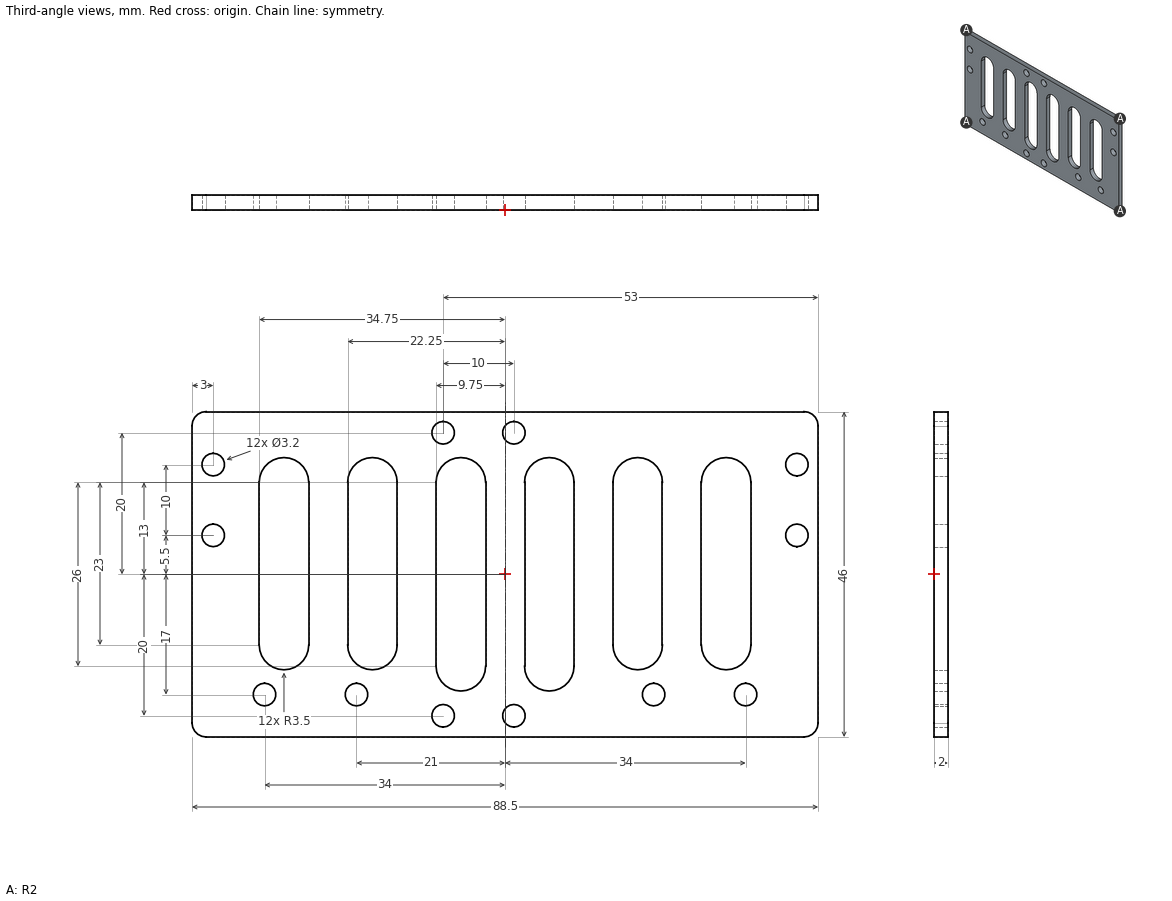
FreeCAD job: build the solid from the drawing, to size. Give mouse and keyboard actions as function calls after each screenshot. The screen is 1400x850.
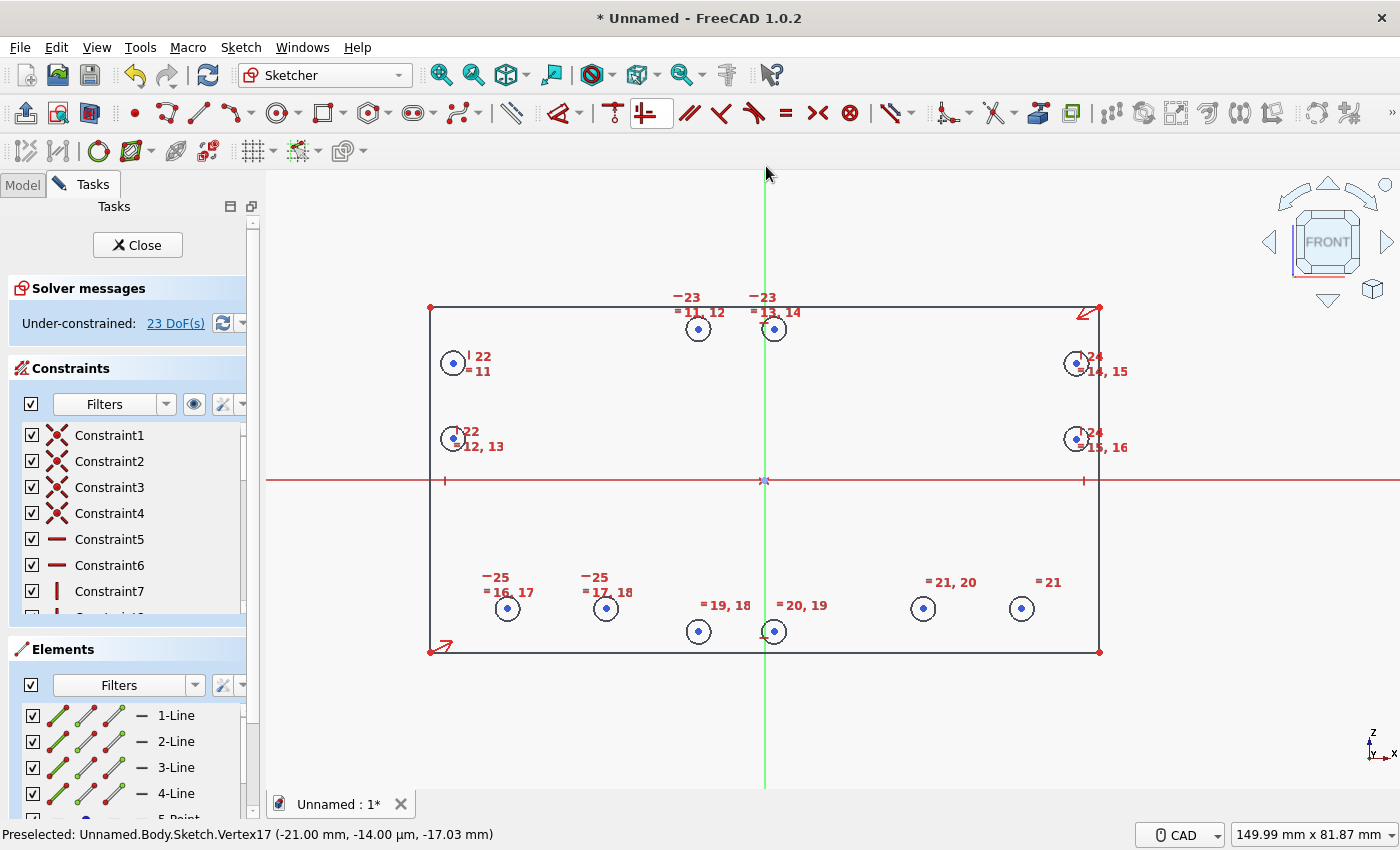
click(698, 329)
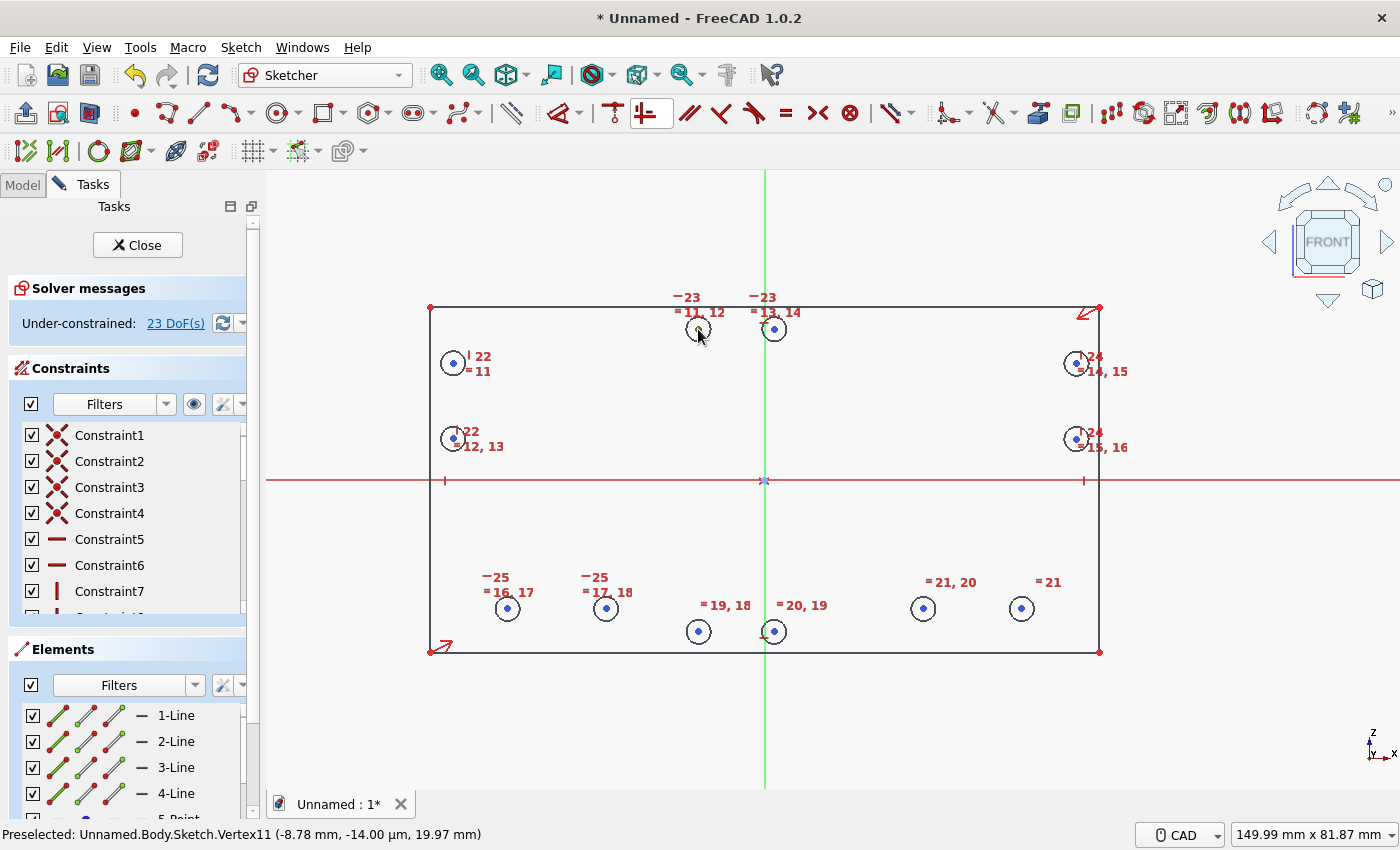
click(699, 632)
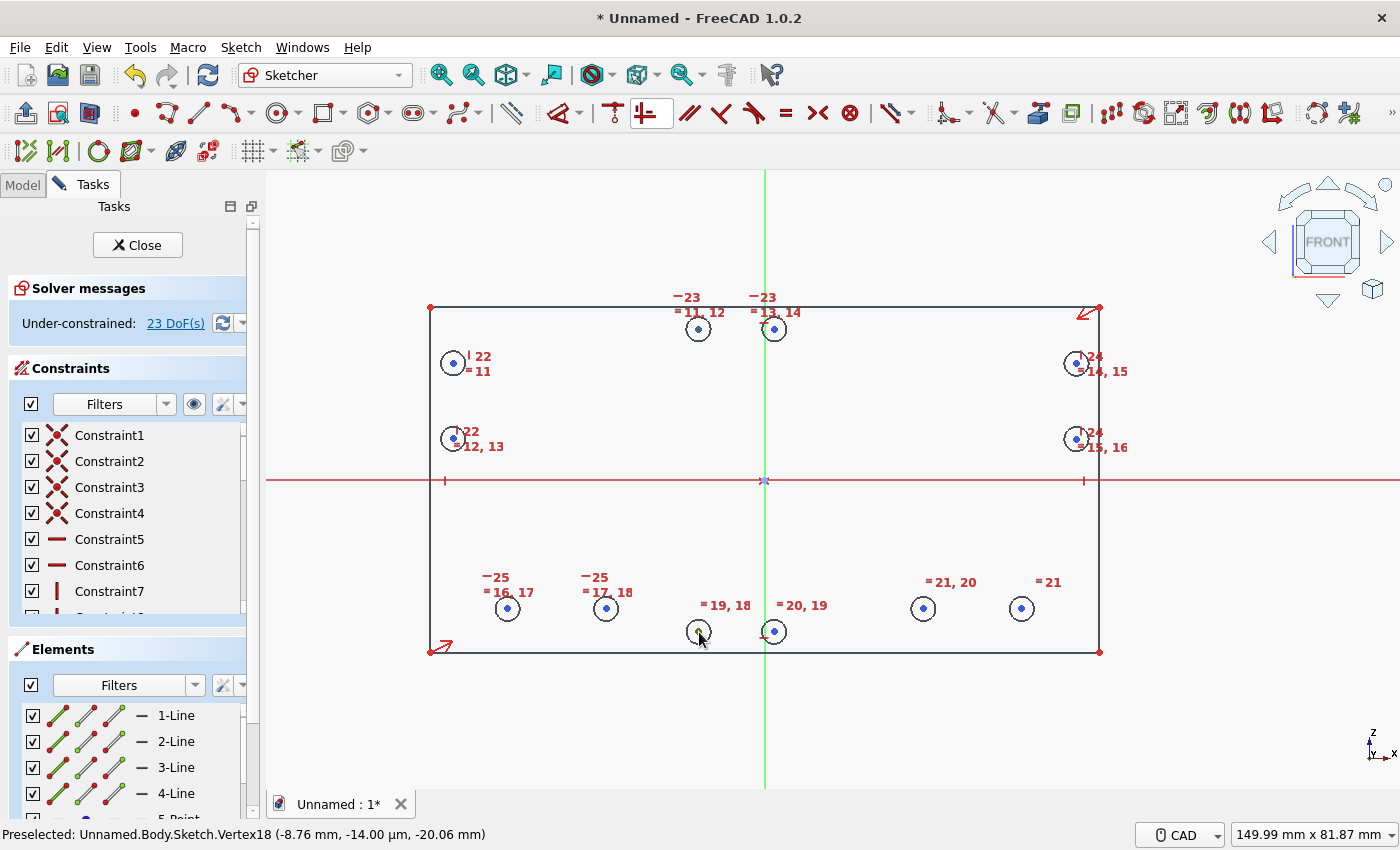
click(668, 114)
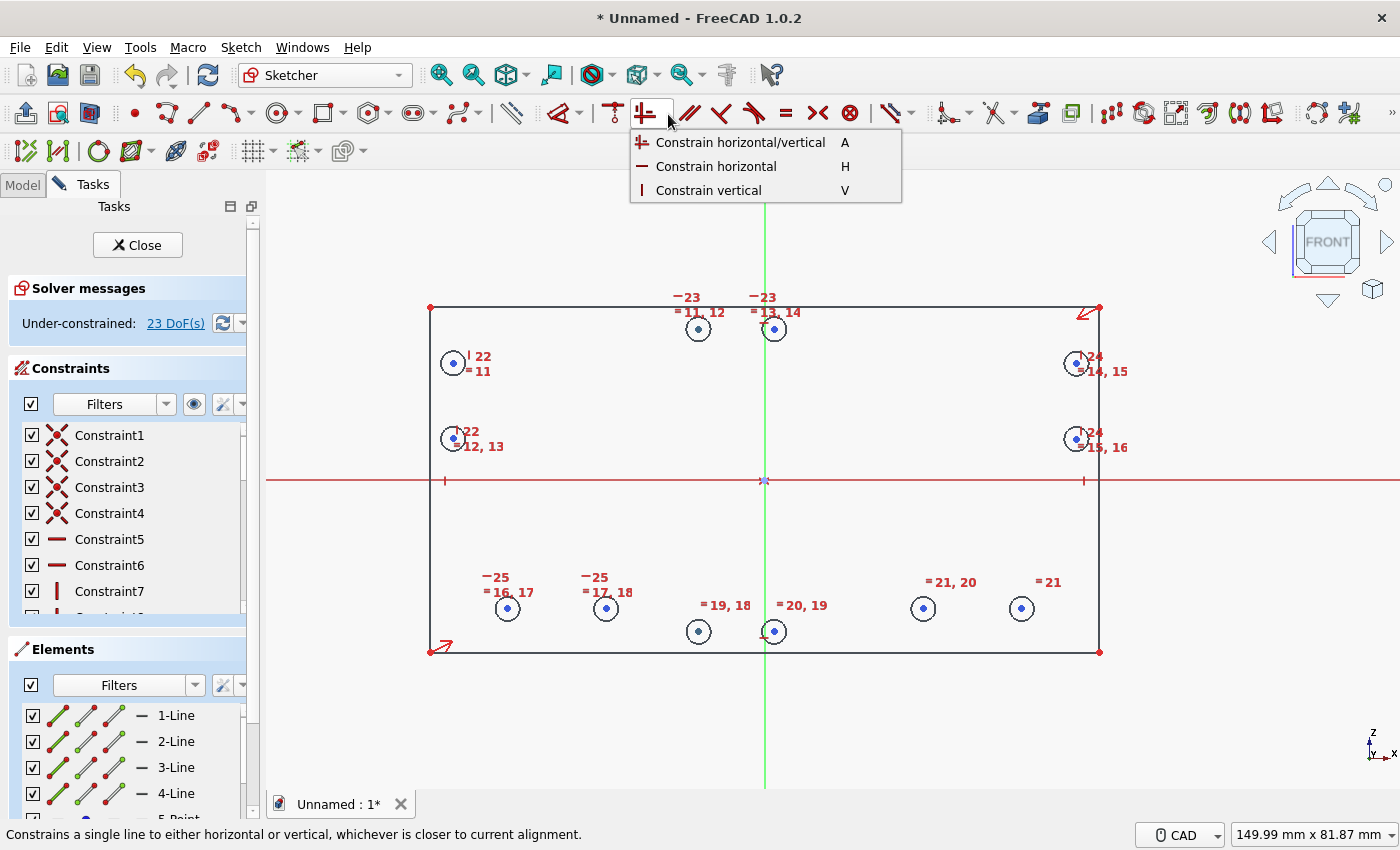
click(766, 190)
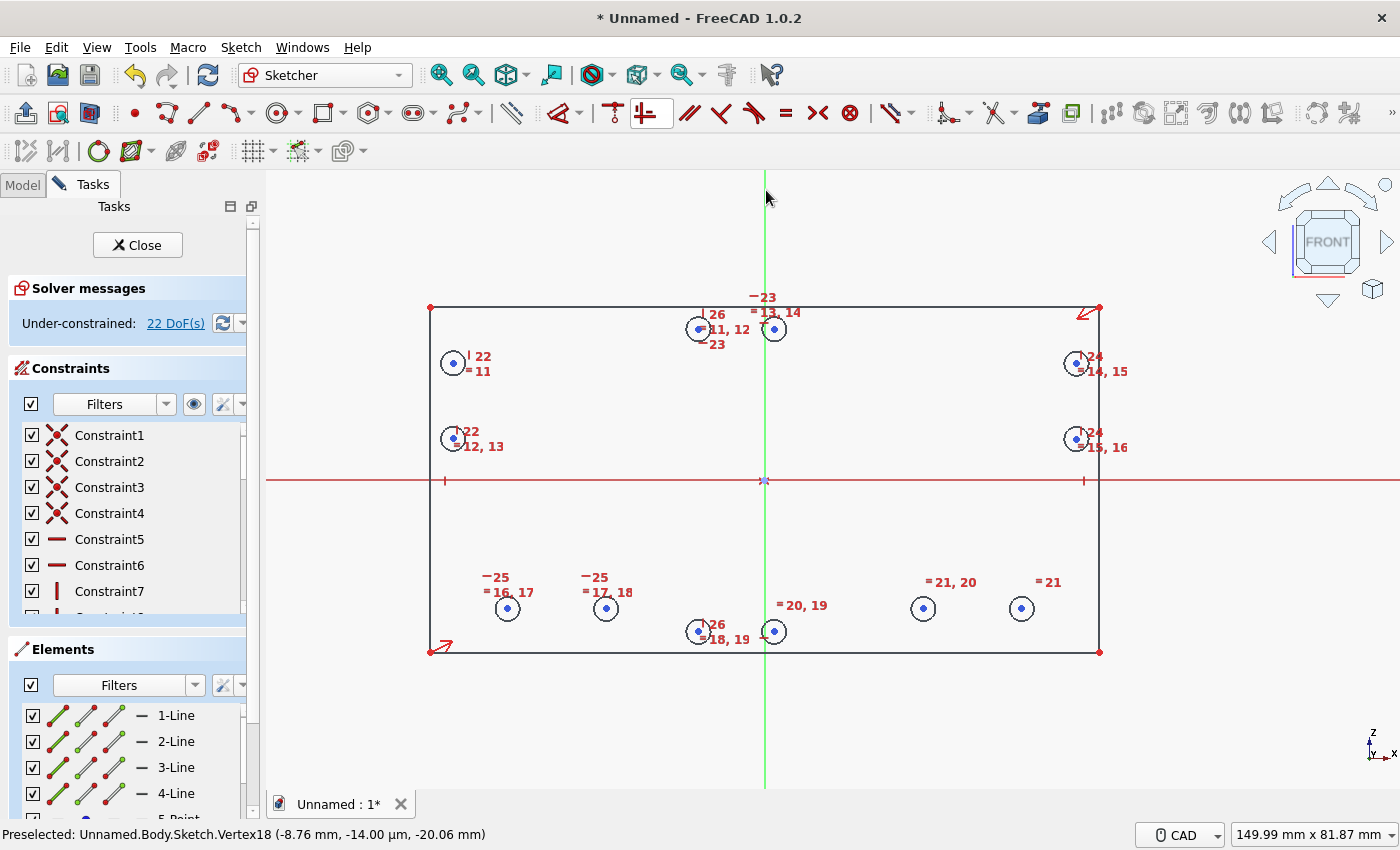
click(774, 329)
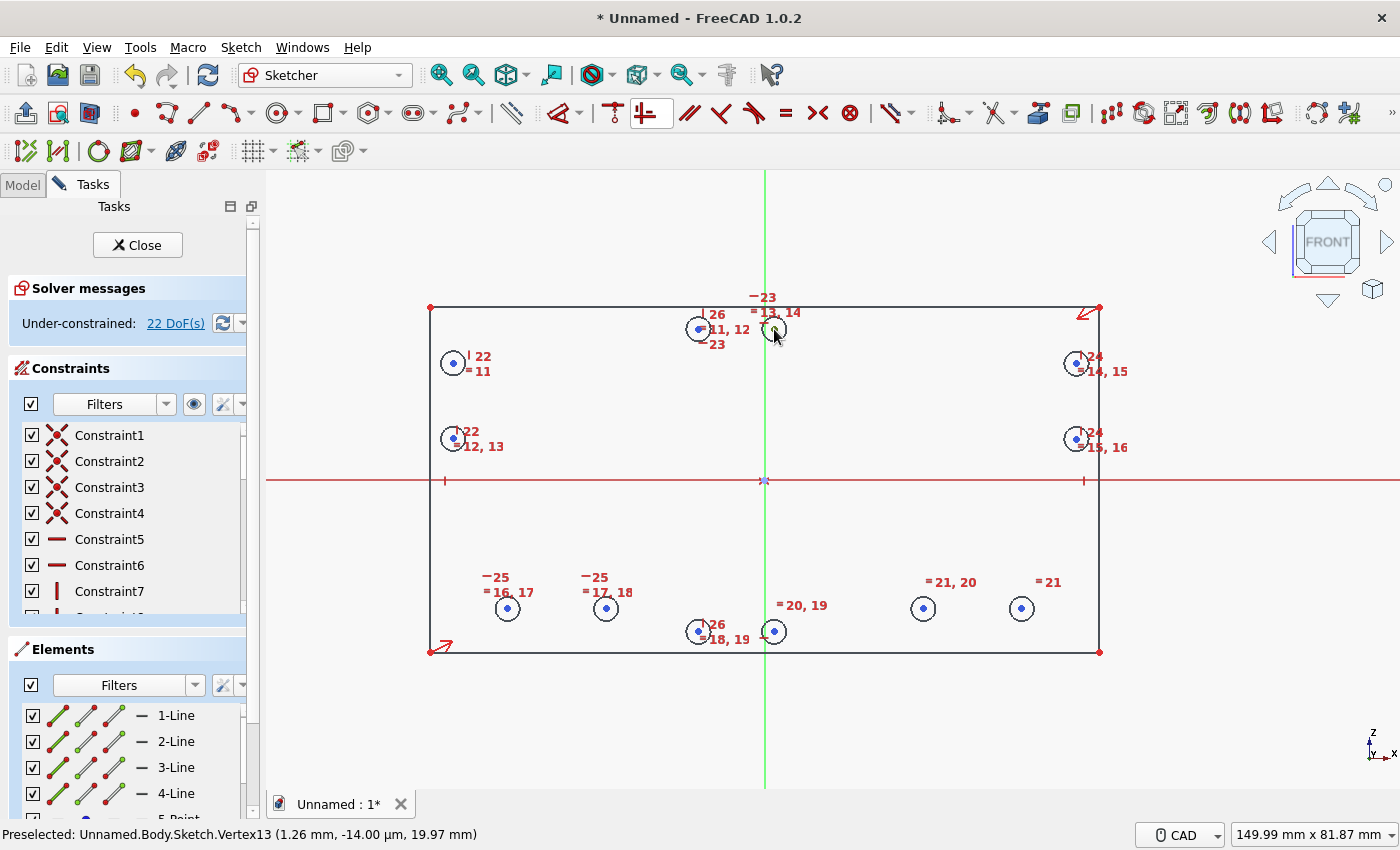
click(774, 632)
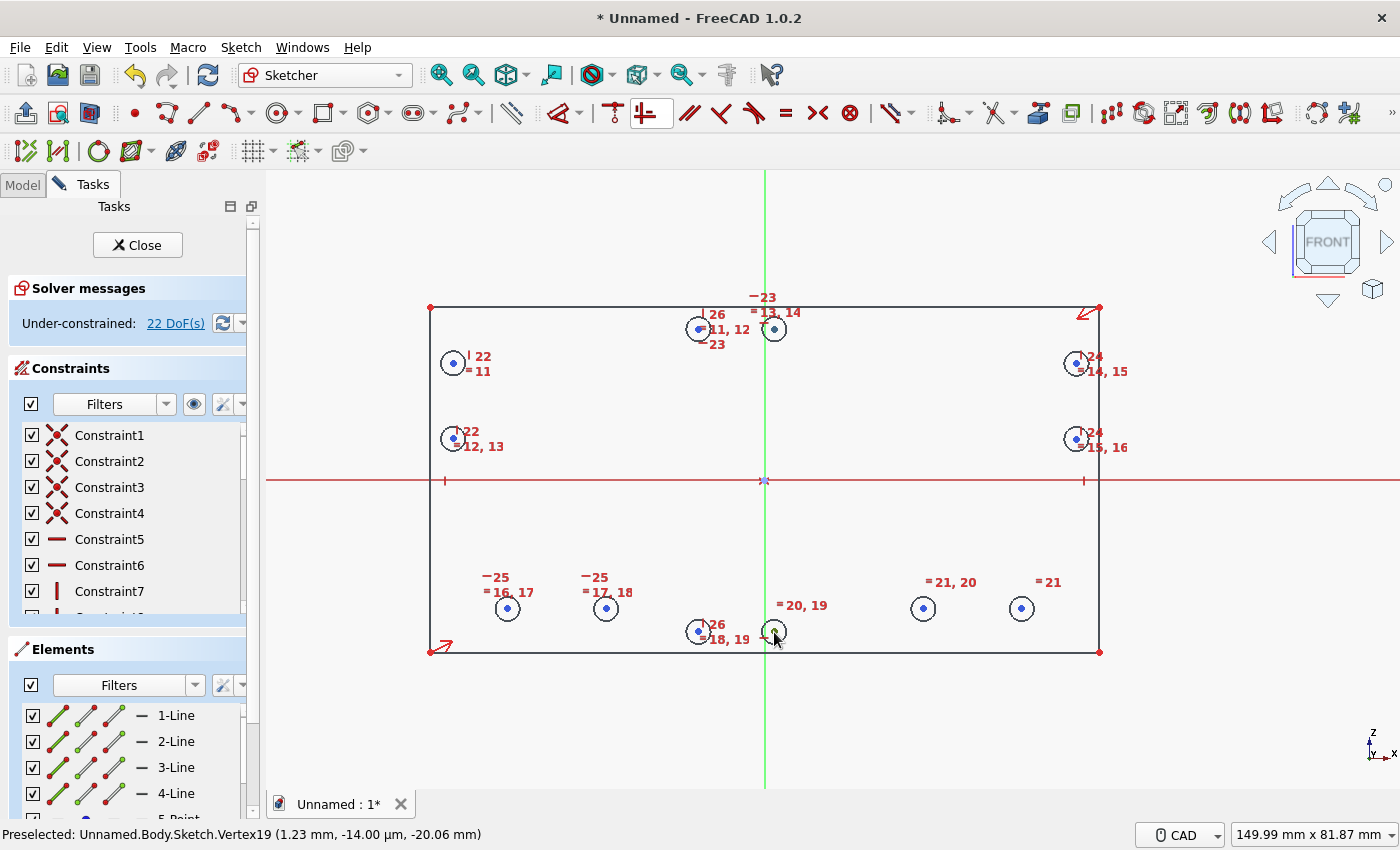
click(668, 114)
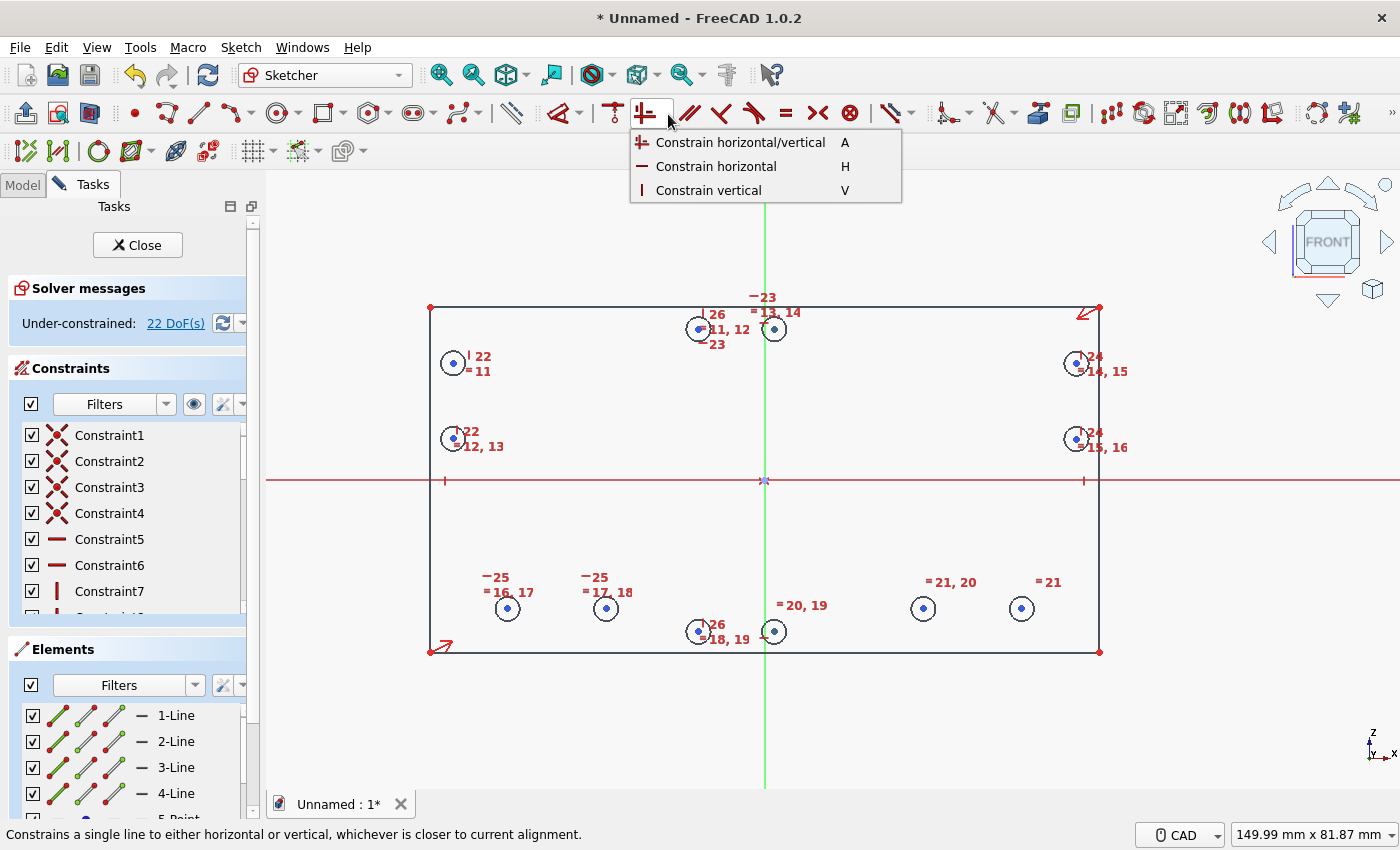
click(766, 190)